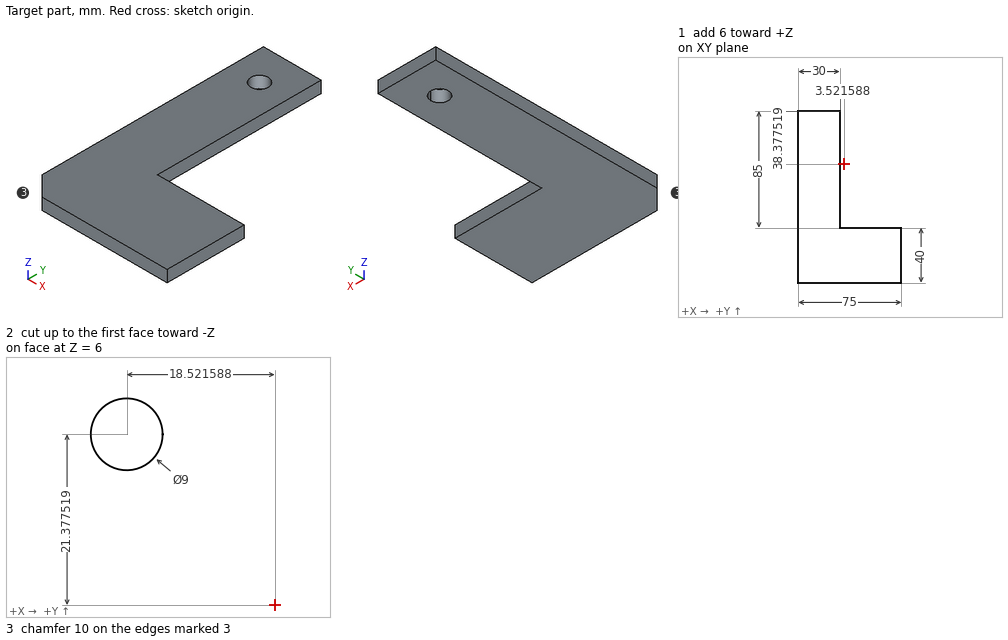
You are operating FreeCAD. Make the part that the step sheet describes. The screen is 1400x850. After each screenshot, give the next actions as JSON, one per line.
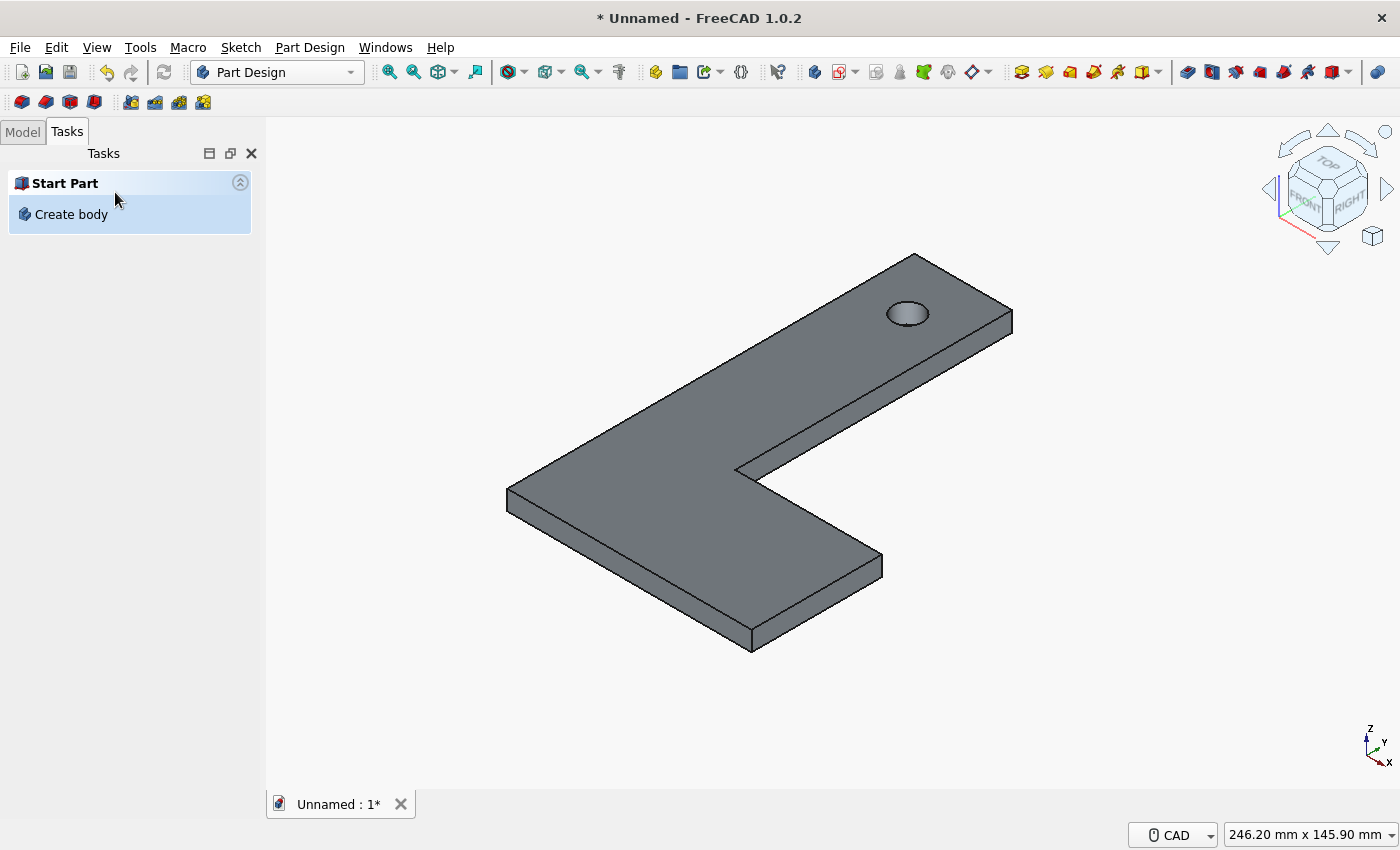
{"action": "key", "text": "2"}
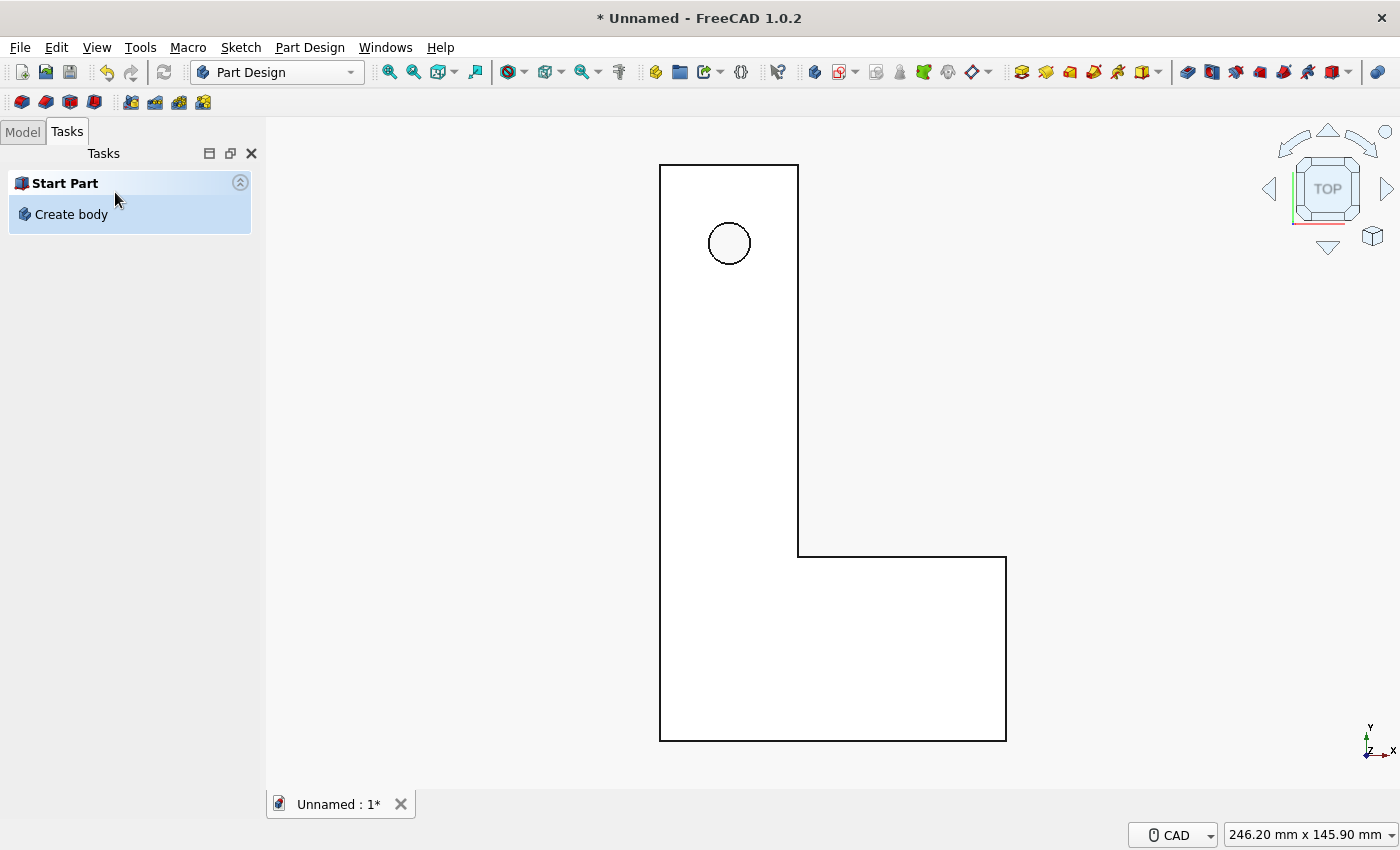
{"action": "key", "text": "1"}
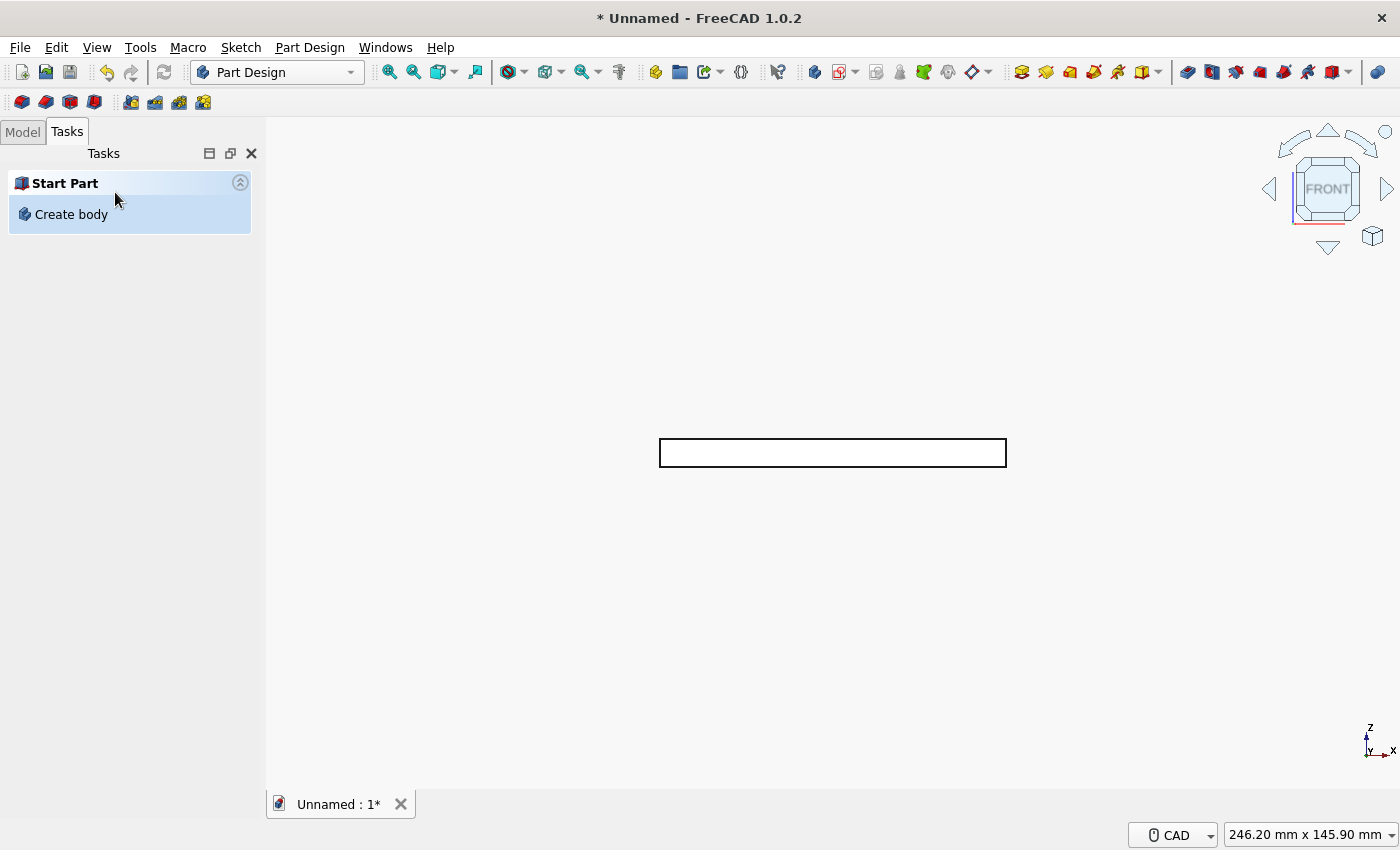
{"action": "left_click", "coordinate": [390, 72]}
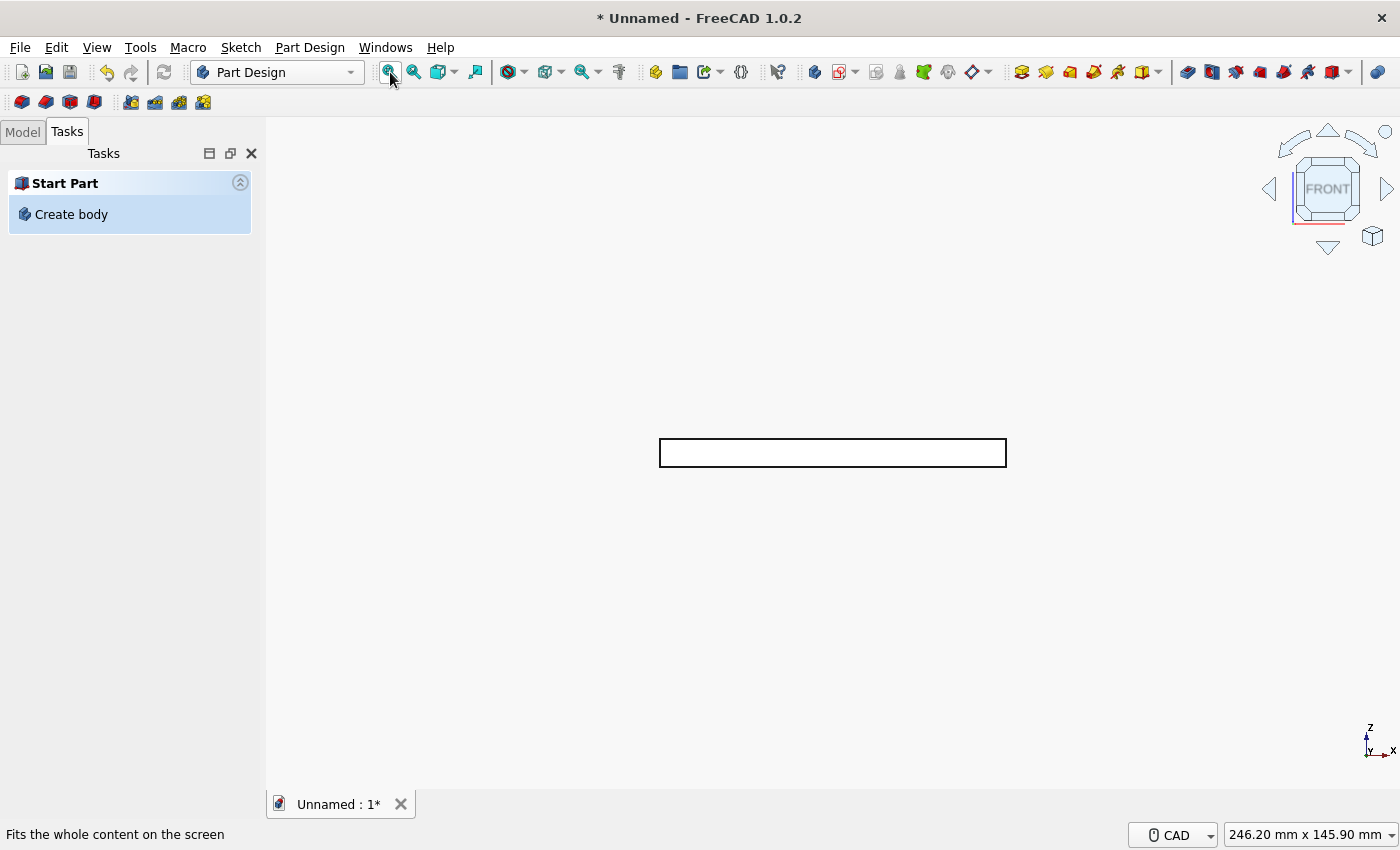
{"action": "left_click", "coordinate": [660, 452]}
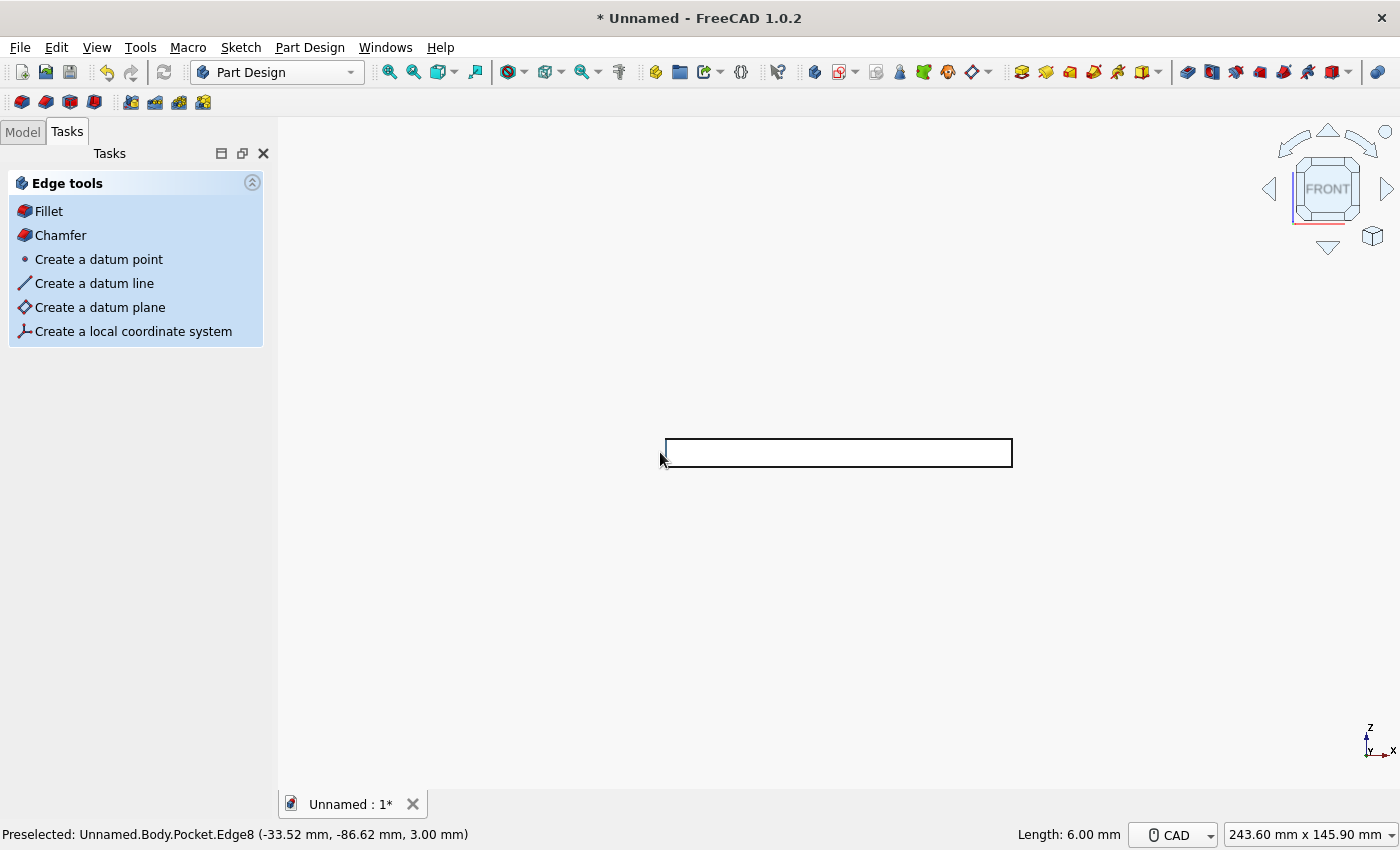
{"action": "left_click", "coordinate": [46, 102]}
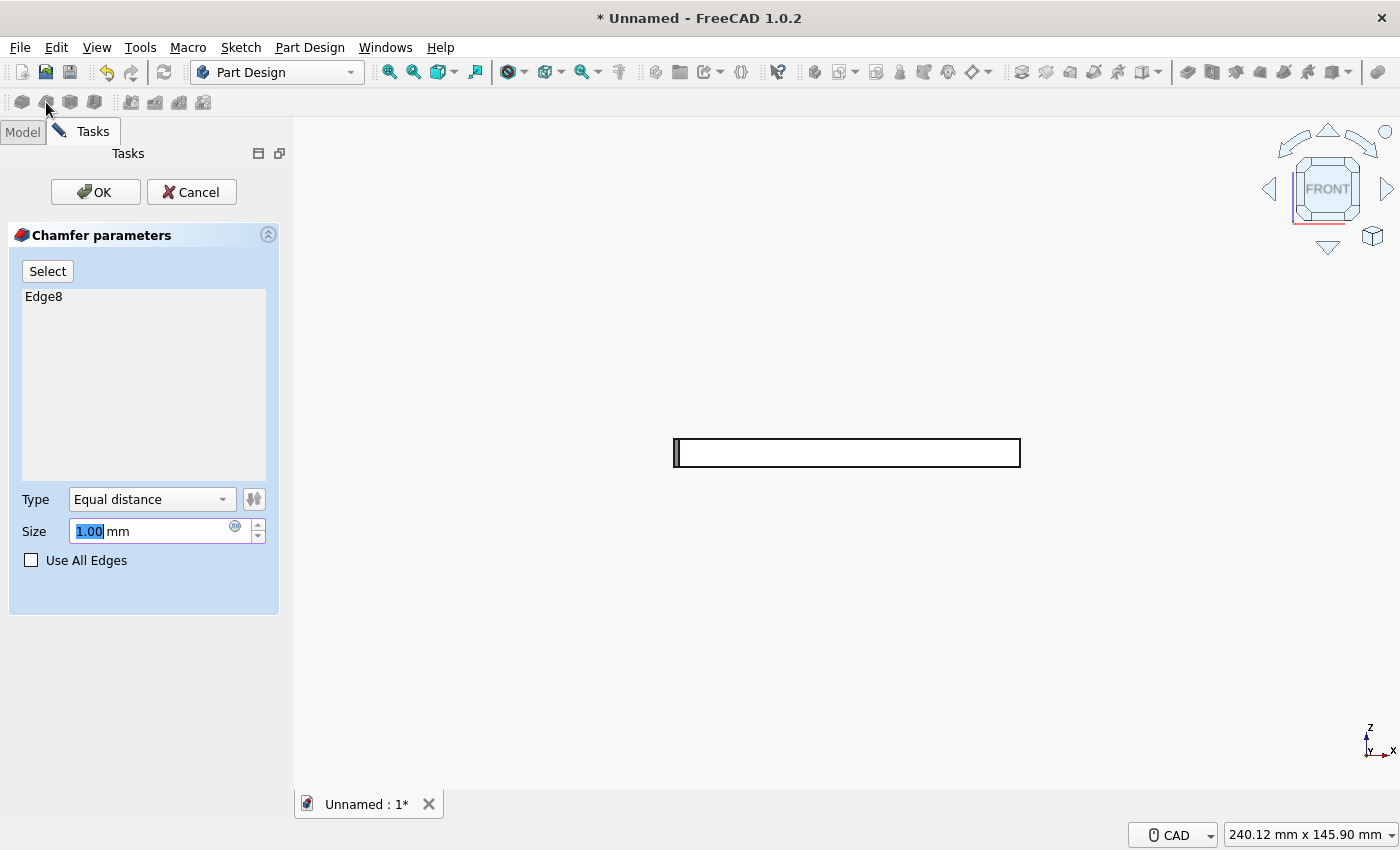
{"action": "type", "text": "10"}
{"action": "key", "text": "Tab"}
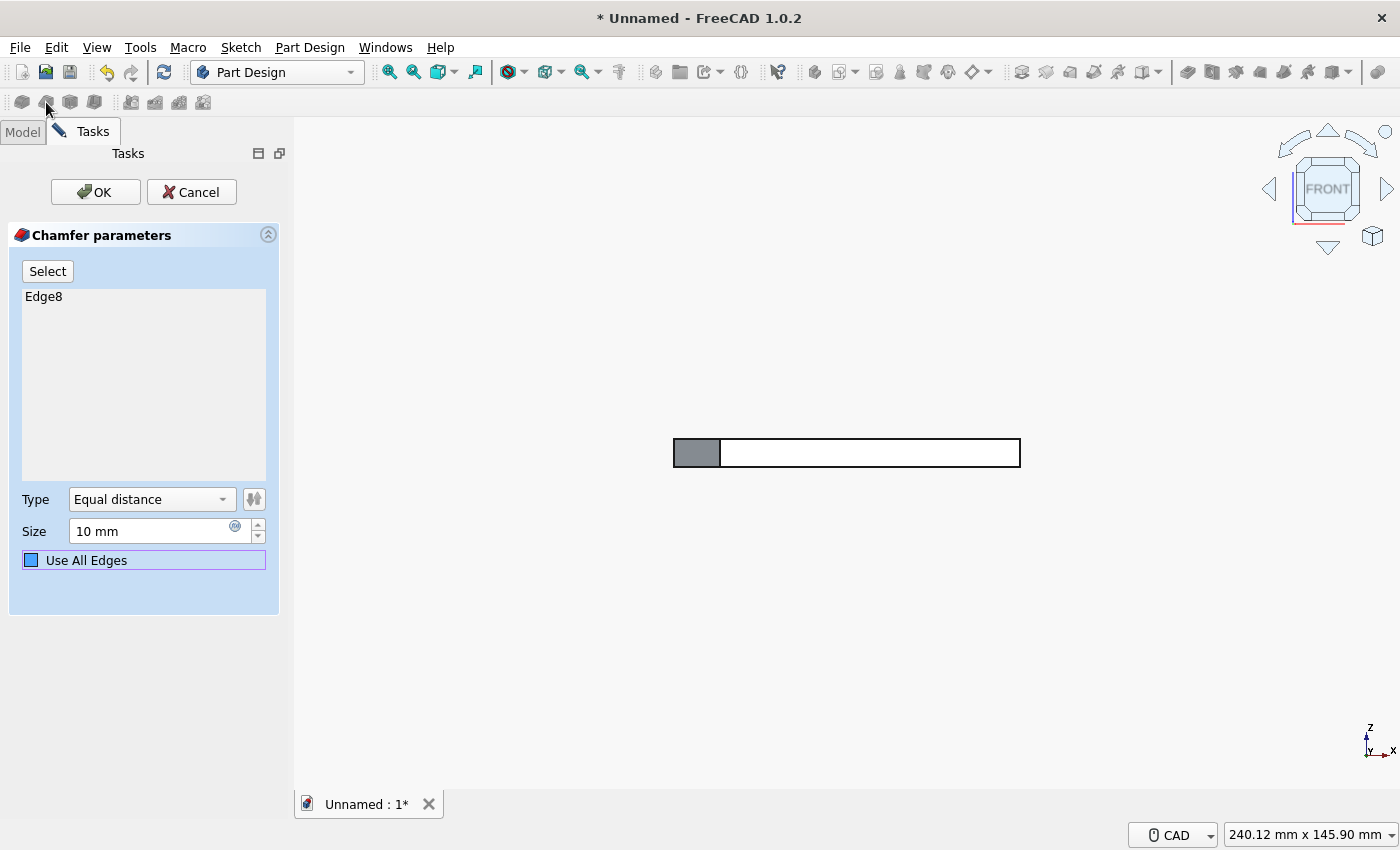
{"action": "left_click", "coordinate": [96, 192]}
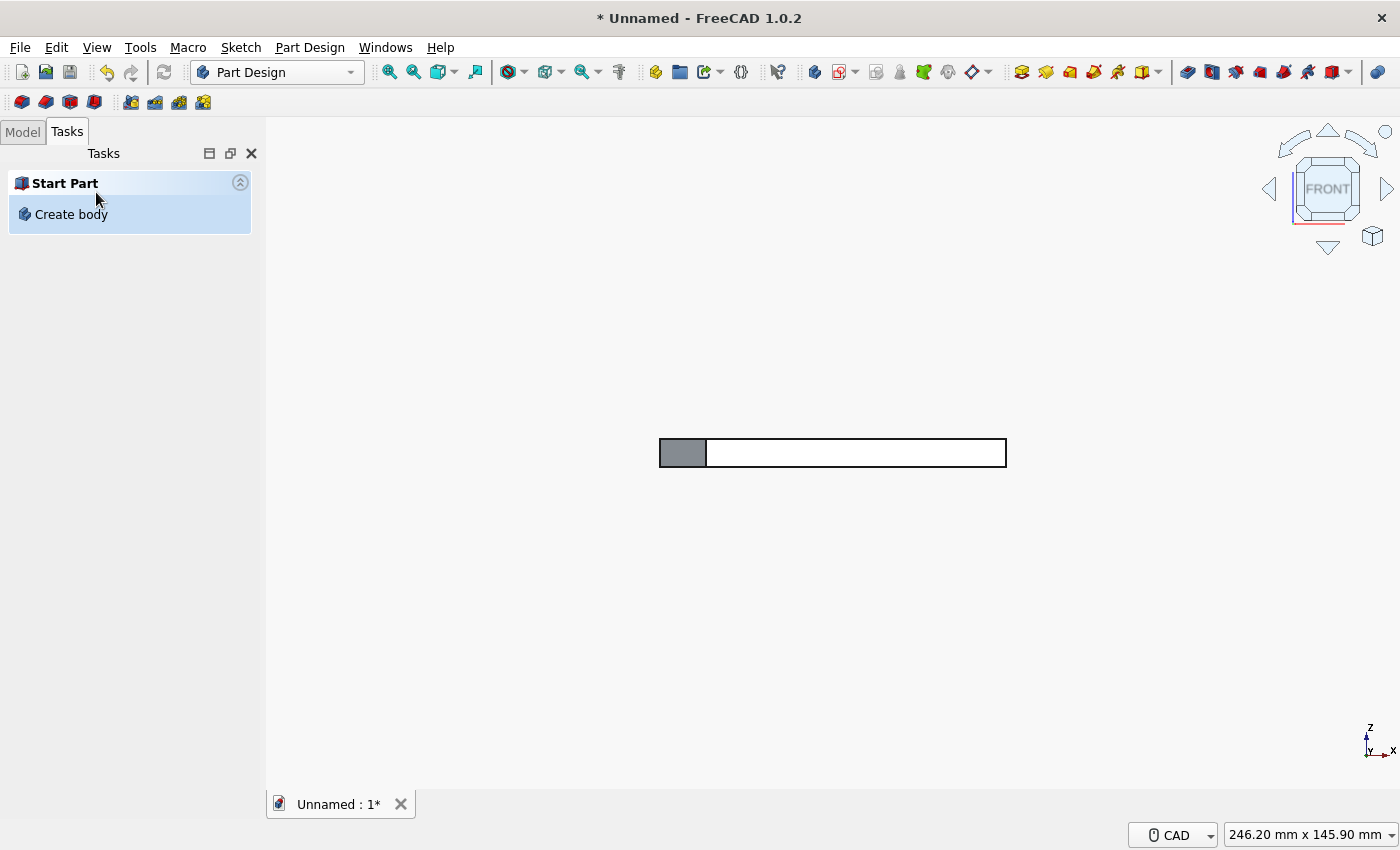
{"action": "key", "text": "0"}